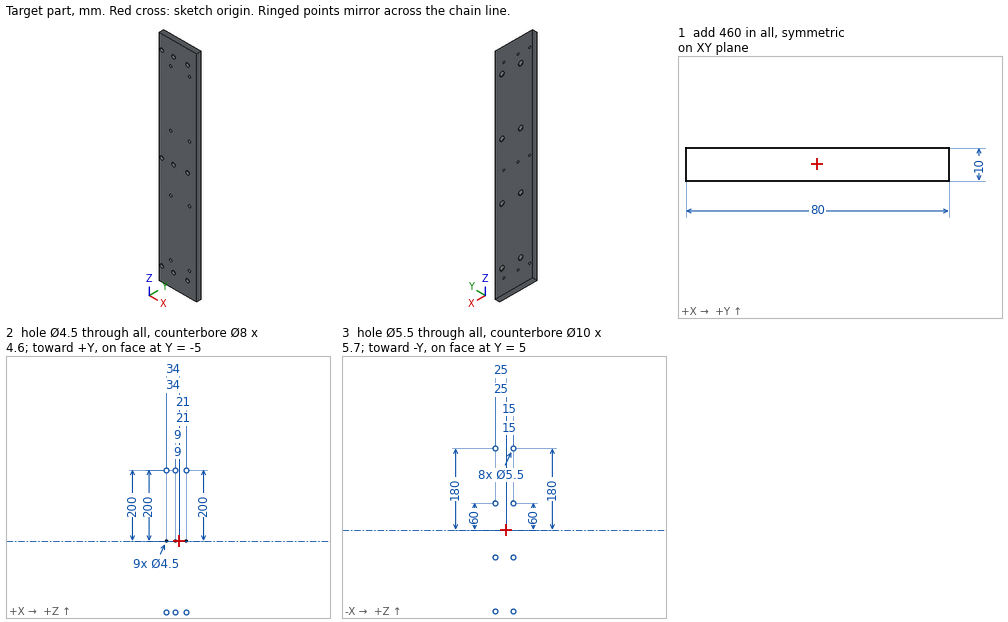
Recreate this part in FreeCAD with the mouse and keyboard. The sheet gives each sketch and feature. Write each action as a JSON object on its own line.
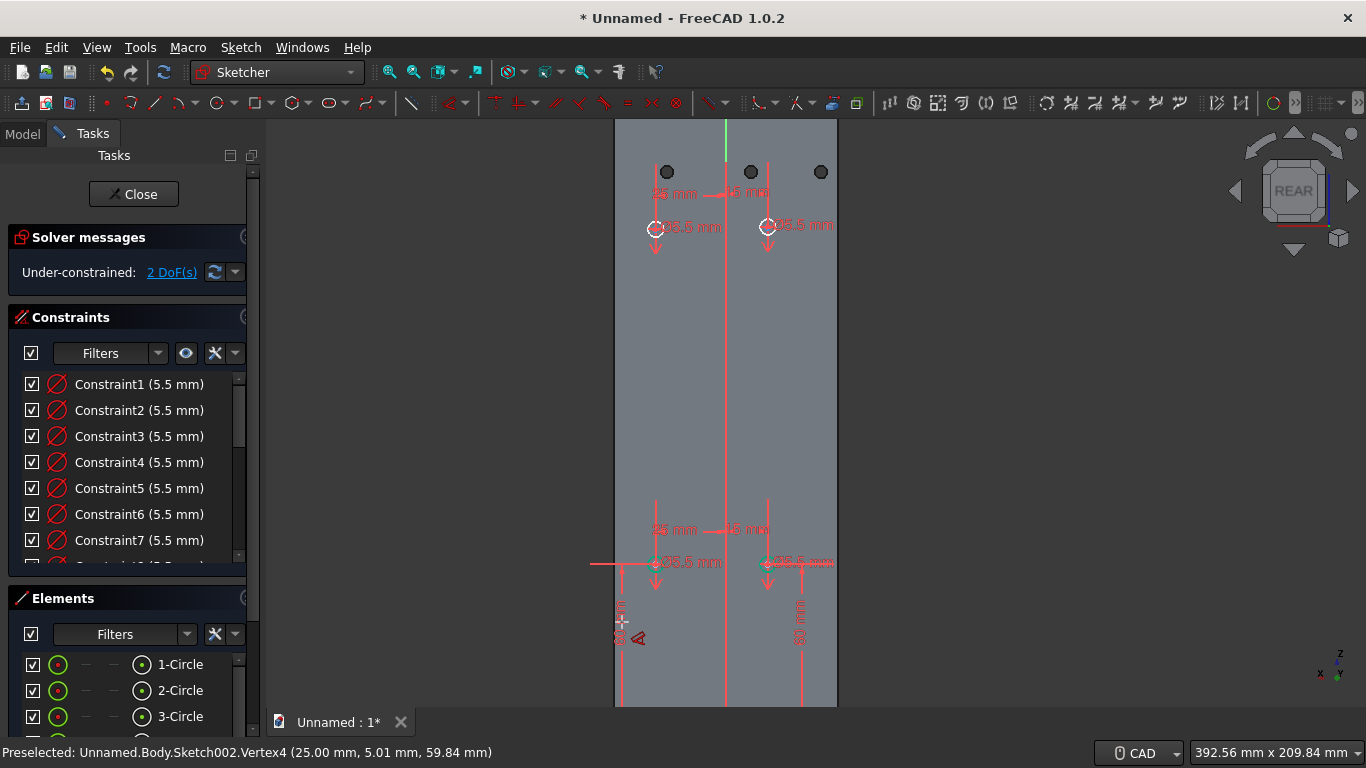
{"action": "left_click", "coordinate": [768, 227]}
{"action": "left_click", "coordinate": [802, 453]}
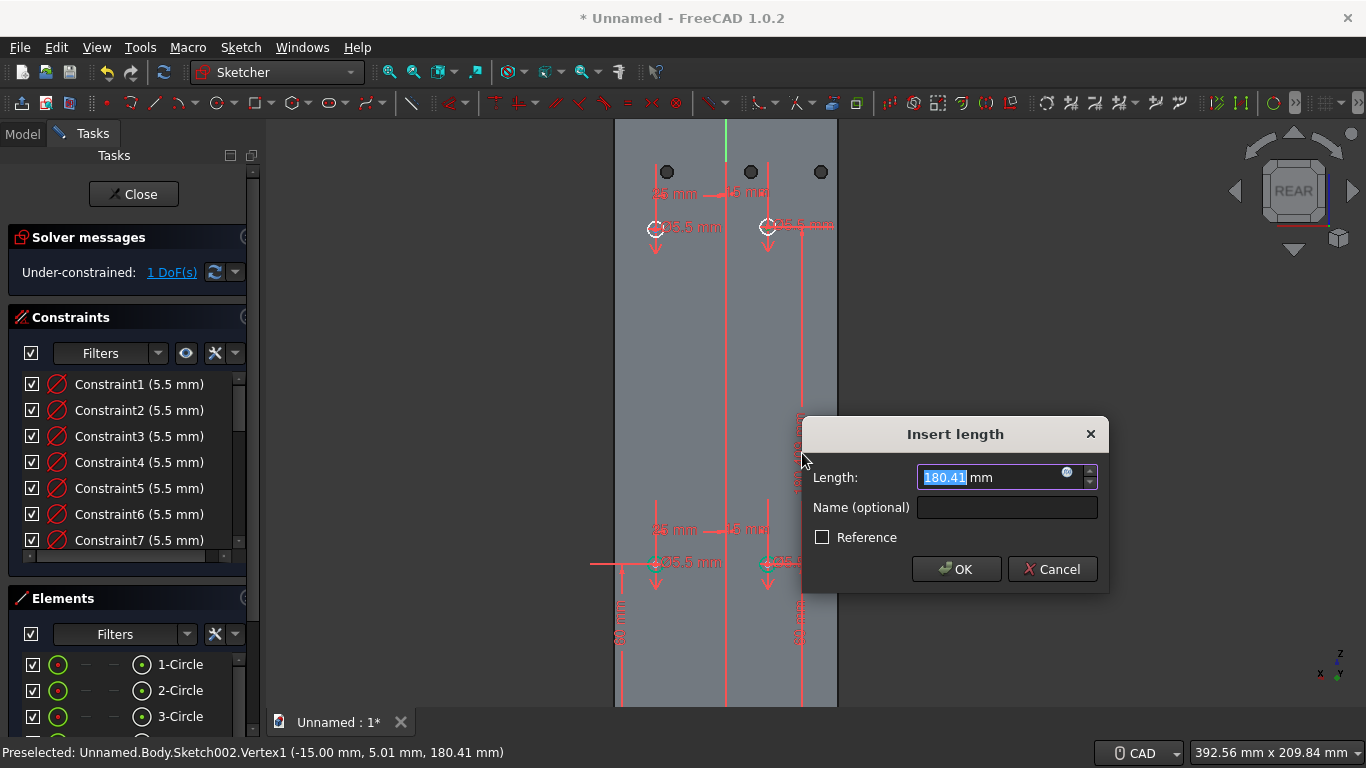
{"action": "type", "text": "180"}
{"action": "key", "text": "Return"}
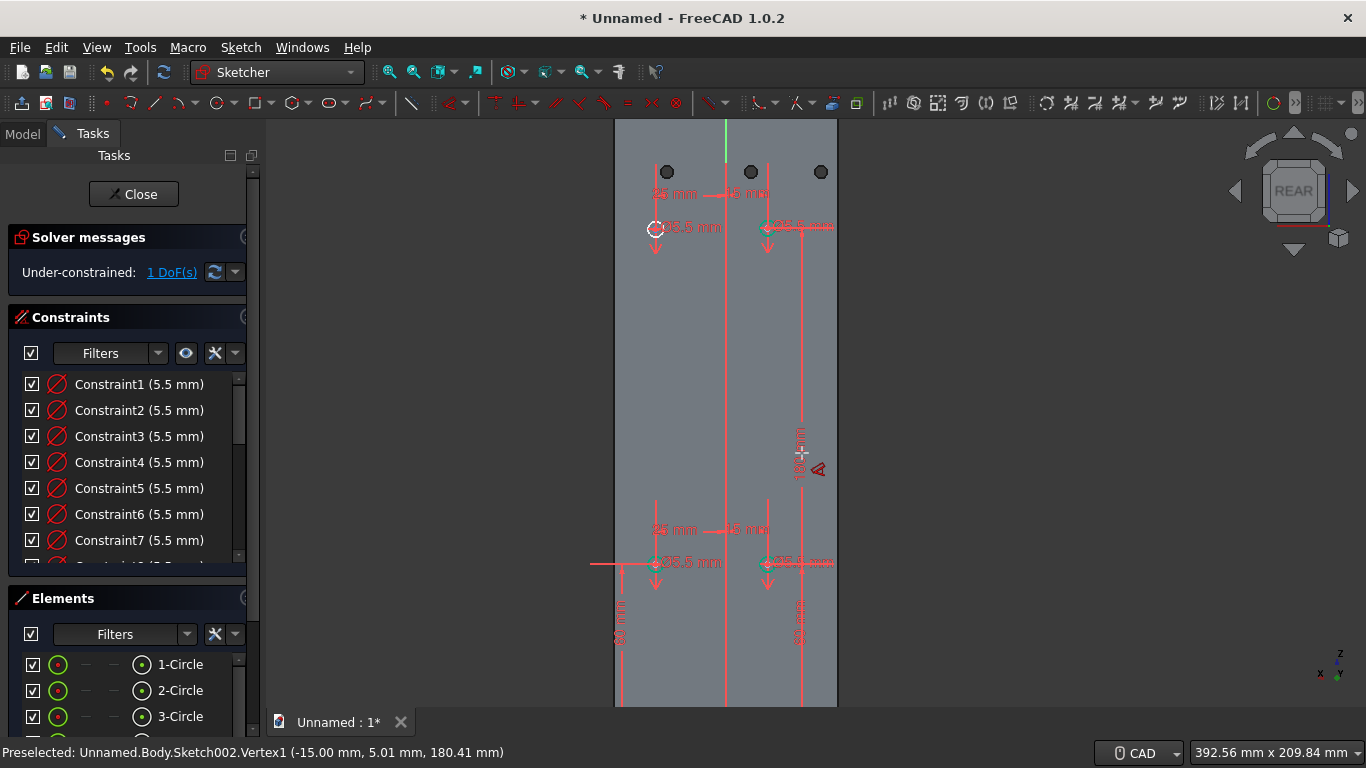
{"action": "left_click", "coordinate": [656, 229]}
{"action": "left_click", "coordinate": [622, 454]}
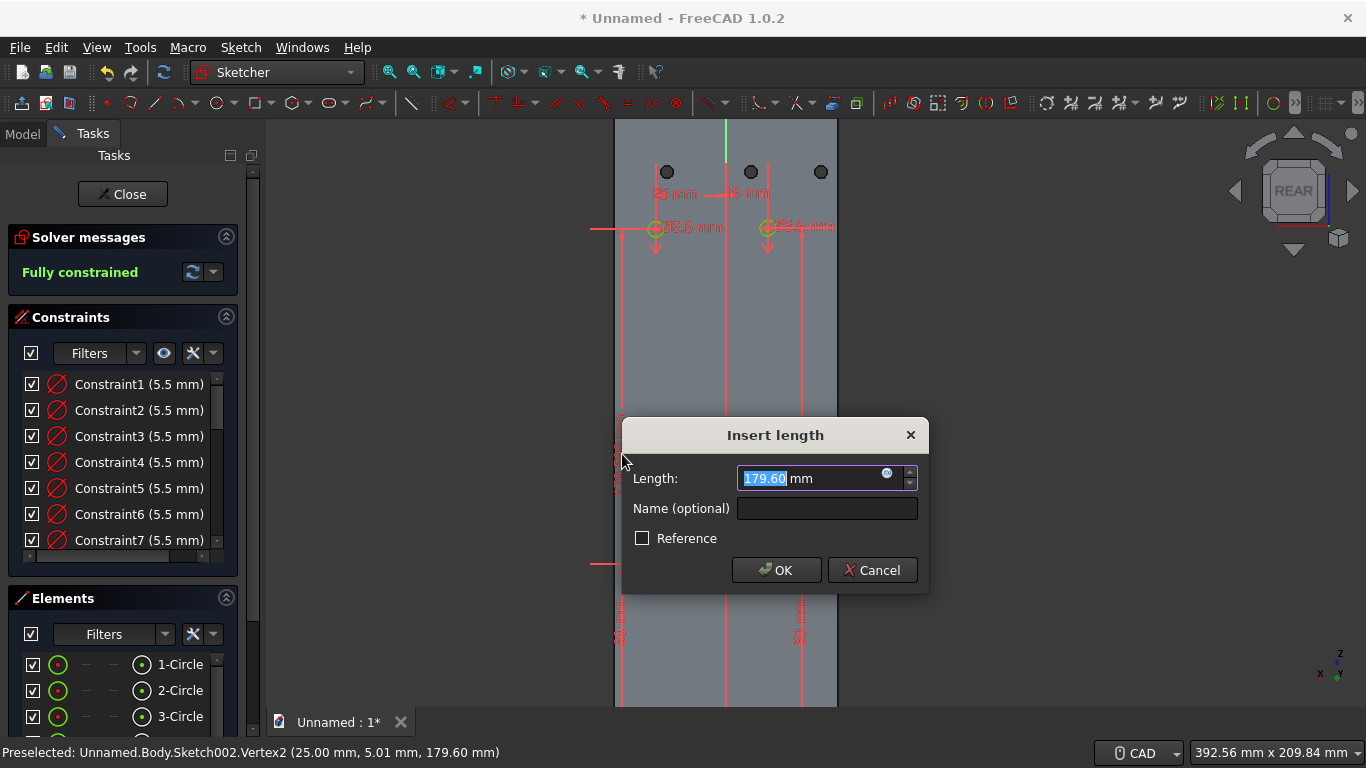
{"action": "type", "text": "180"}
{"action": "key", "text": "Return"}
{"action": "key", "text": "Escape"}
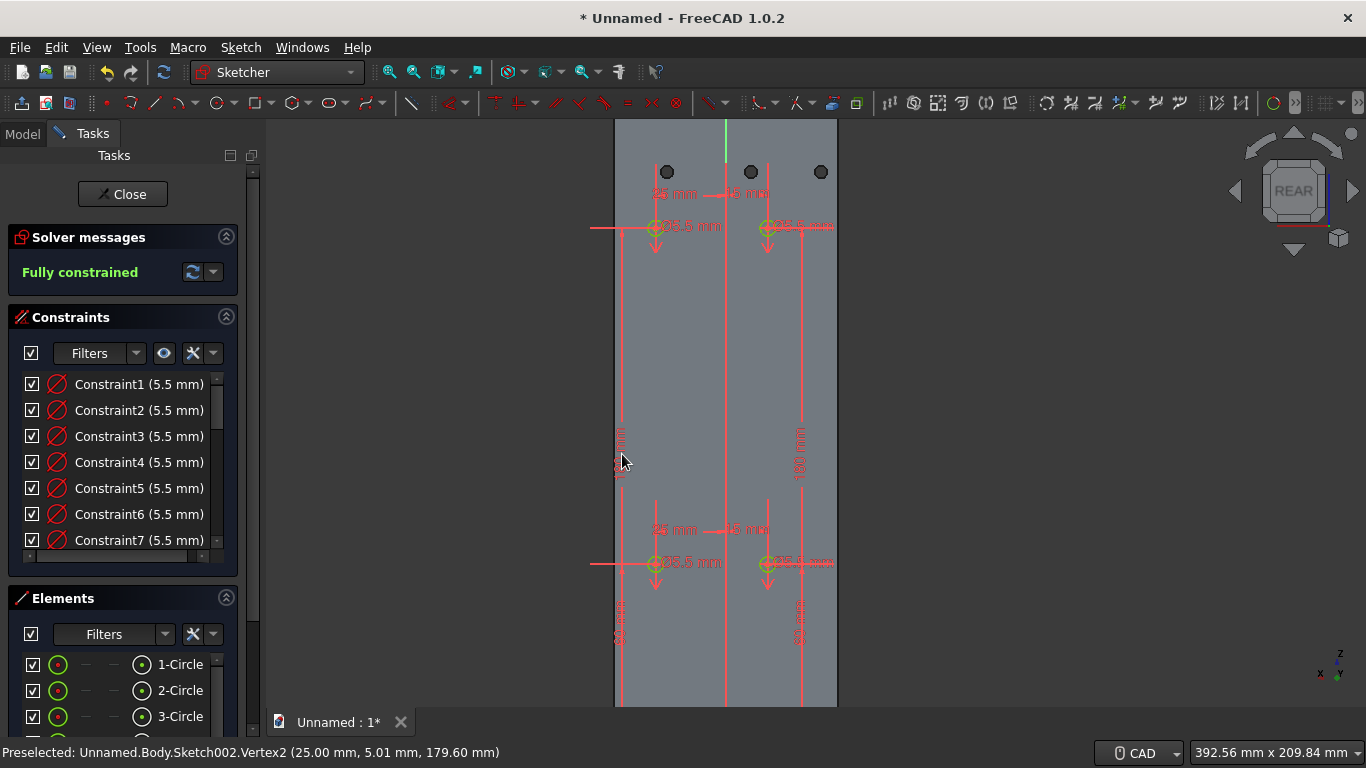
{"action": "left_click", "coordinate": [123, 194]}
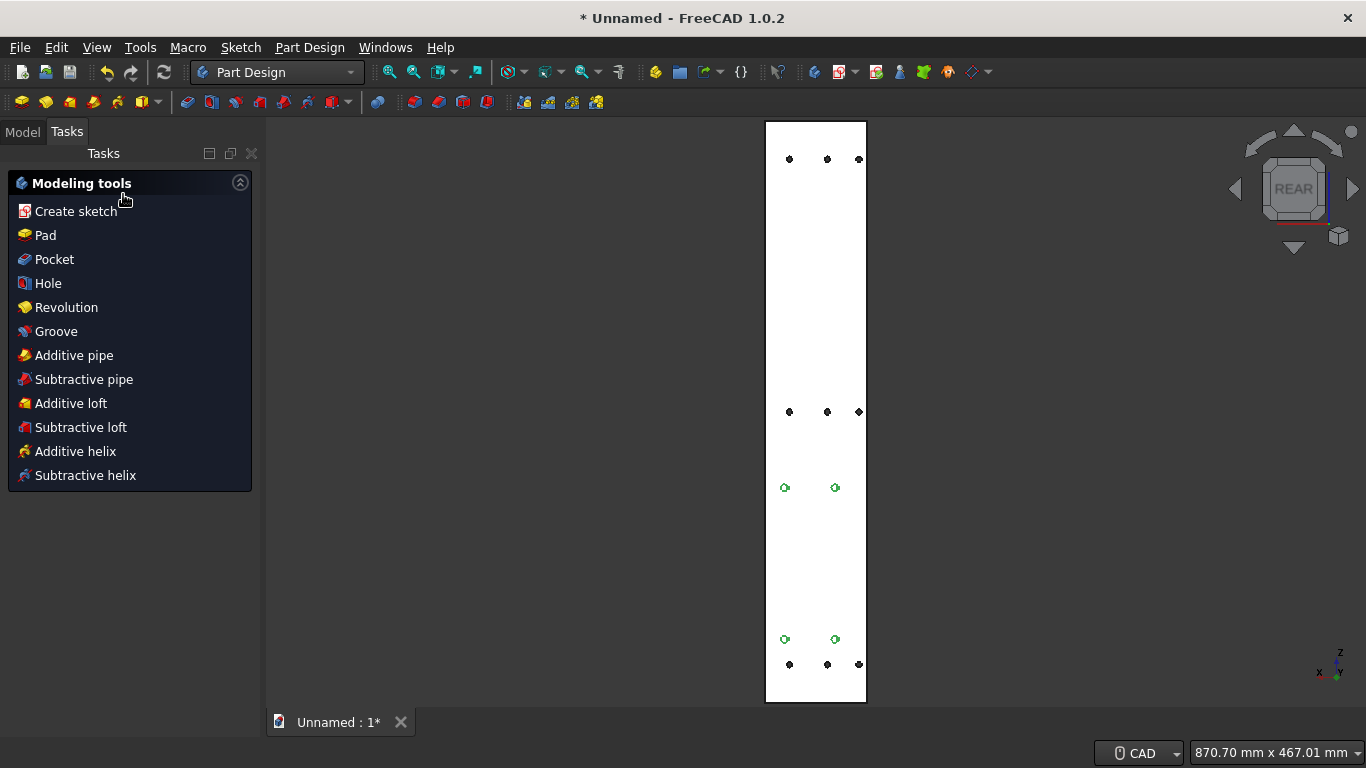
{"action": "left_click", "coordinate": [212, 102]}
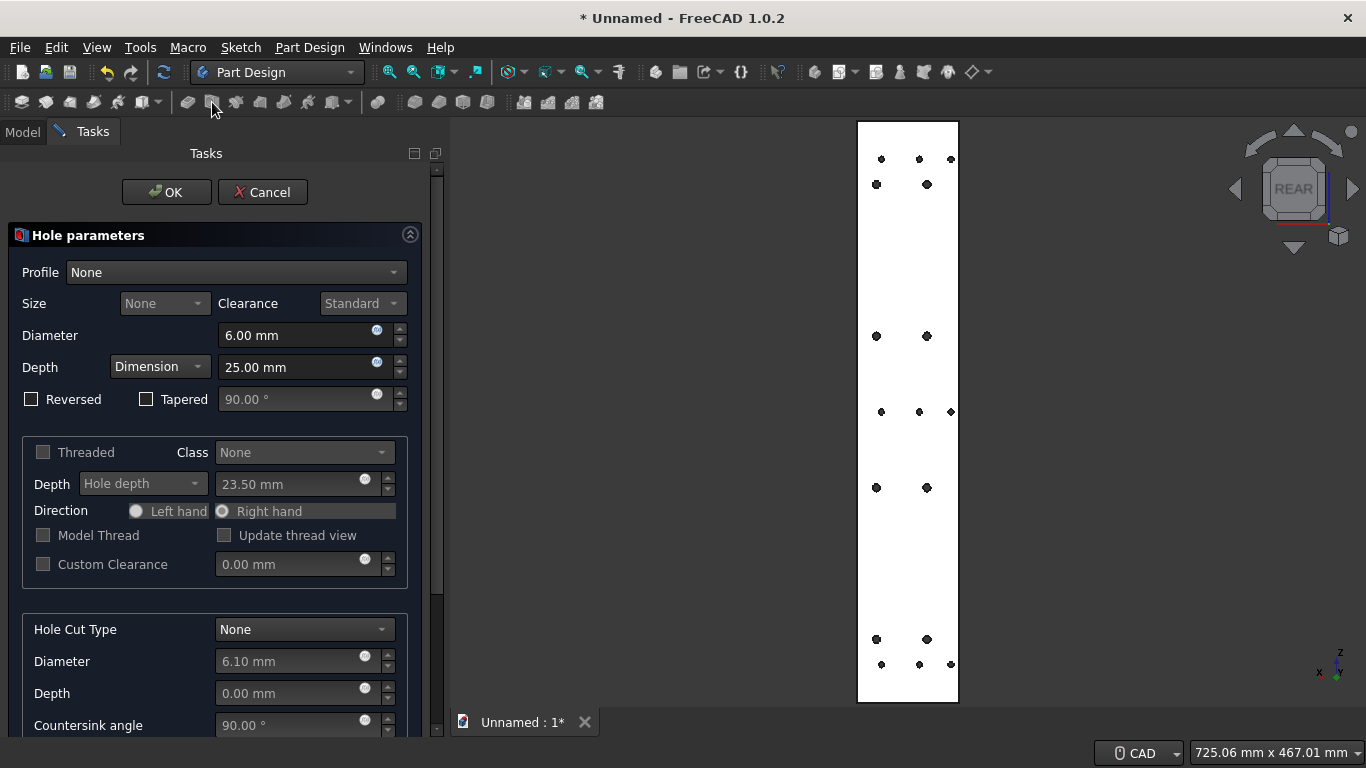
{"action": "triple_click", "coordinate": [305, 335]}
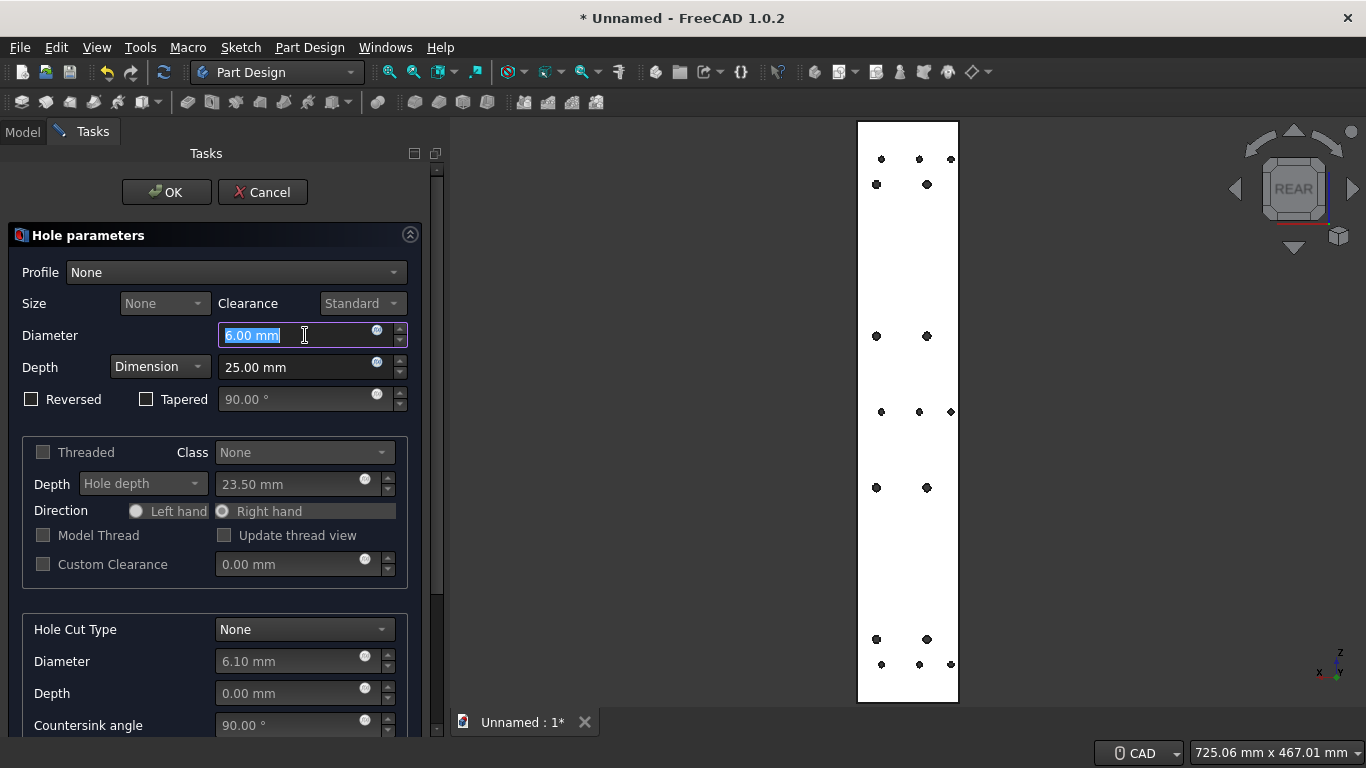
{"action": "type", "text": "5.5"}
{"action": "key", "text": "Tab"}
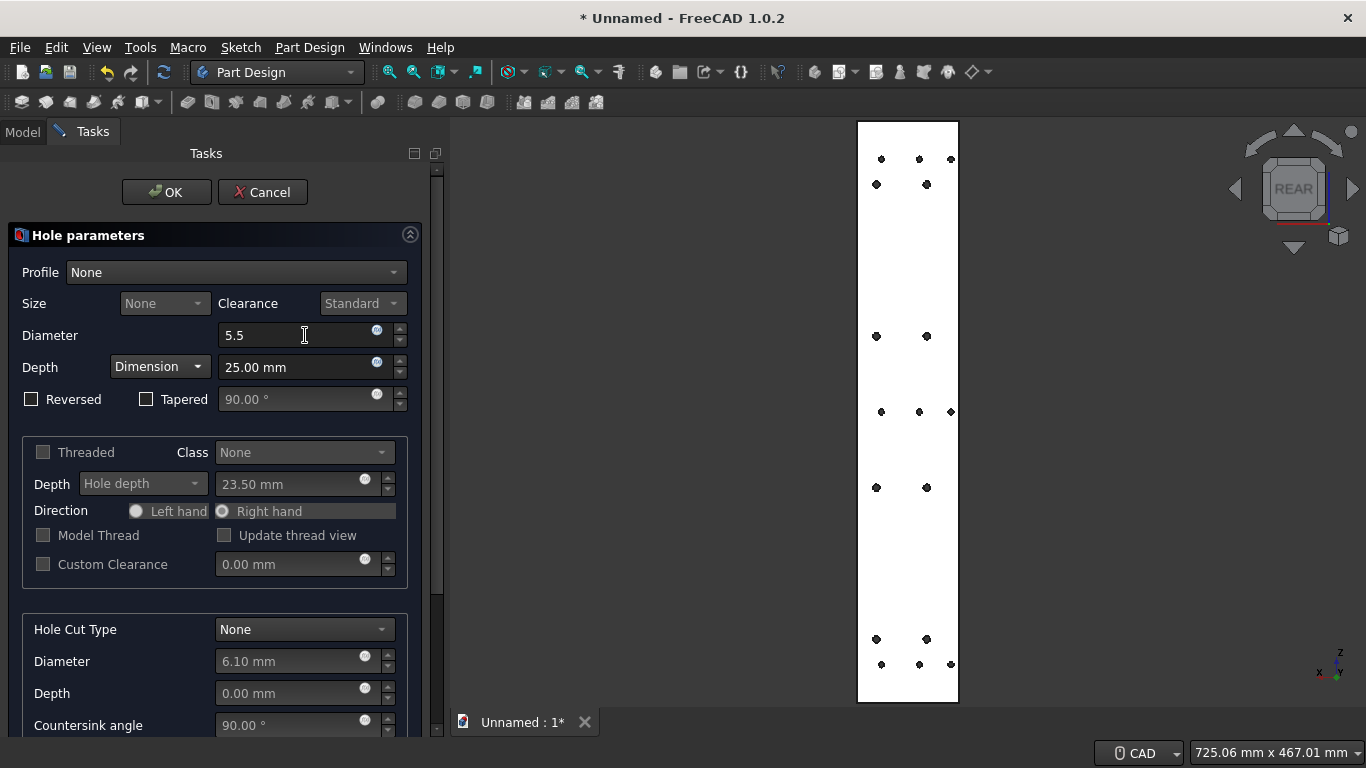
{"action": "left_click", "coordinate": [161, 366]}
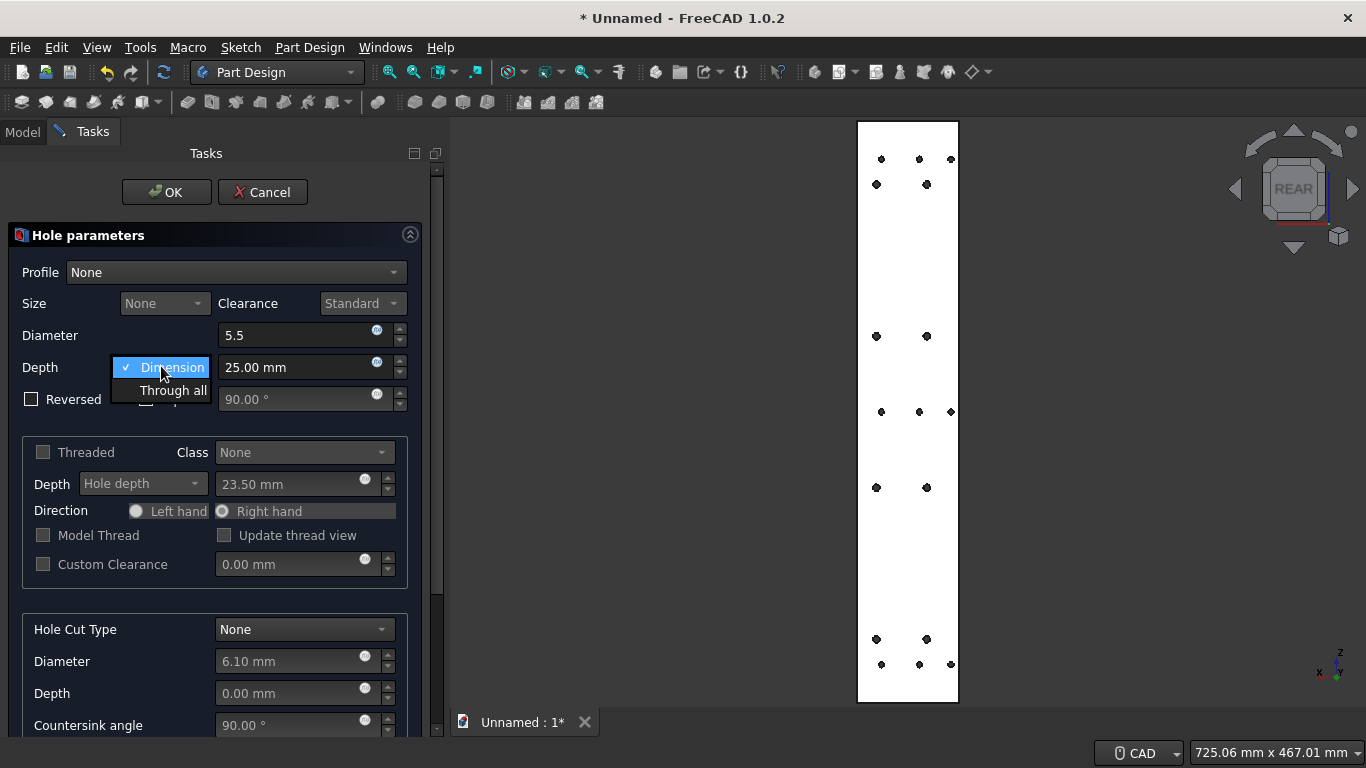
{"action": "left_click", "coordinate": [160, 390]}